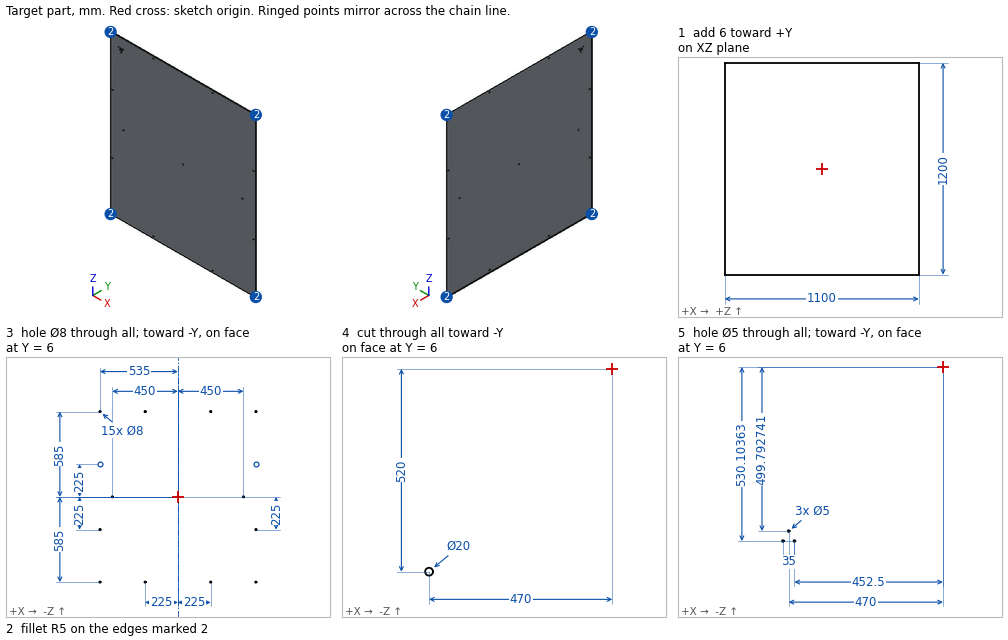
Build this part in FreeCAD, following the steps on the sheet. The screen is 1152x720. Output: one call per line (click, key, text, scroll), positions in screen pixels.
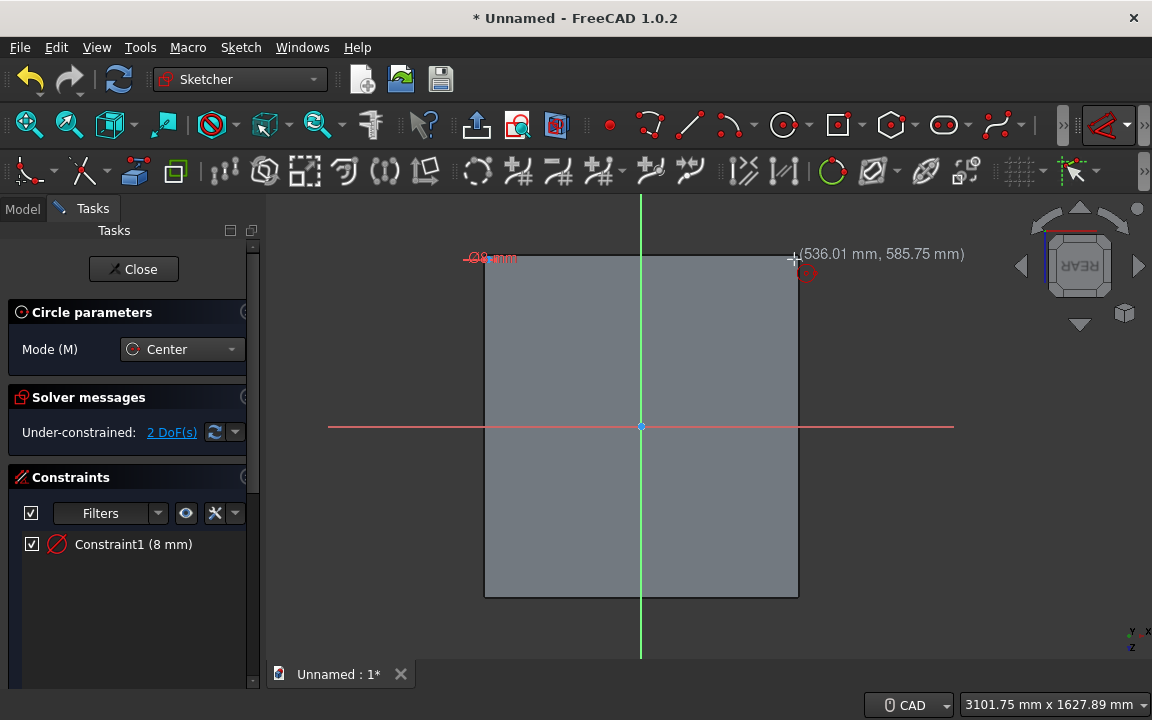
click(794, 259)
move(795, 259)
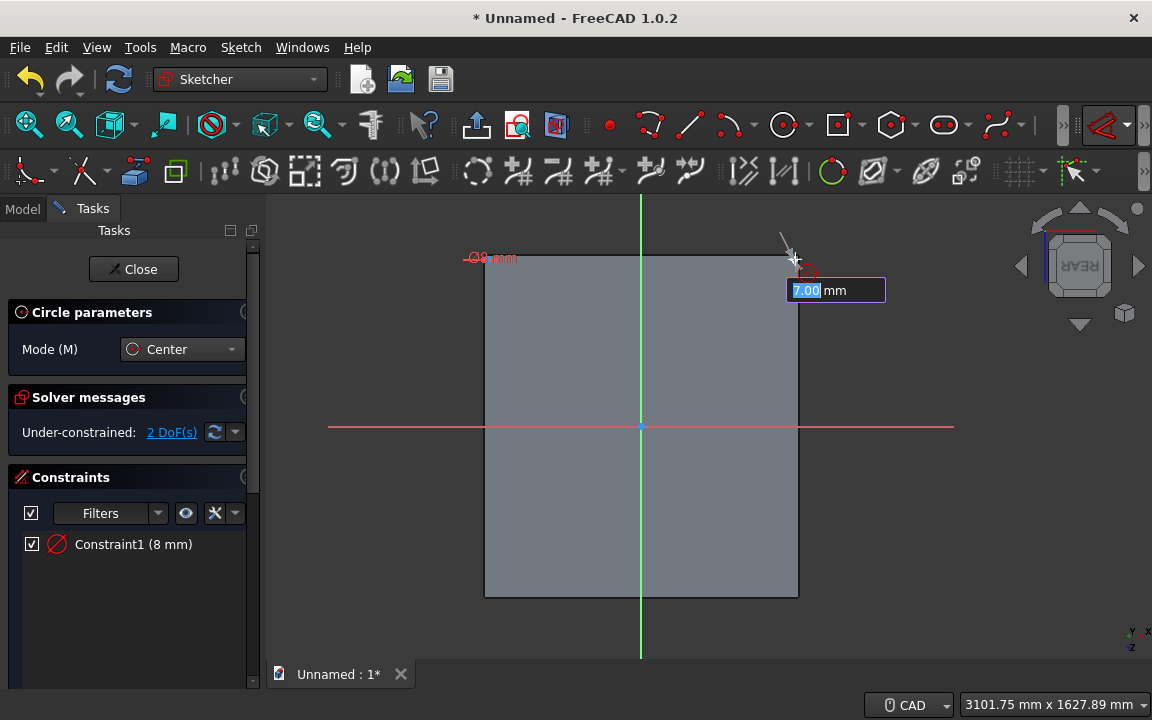
text(8)
key(Return)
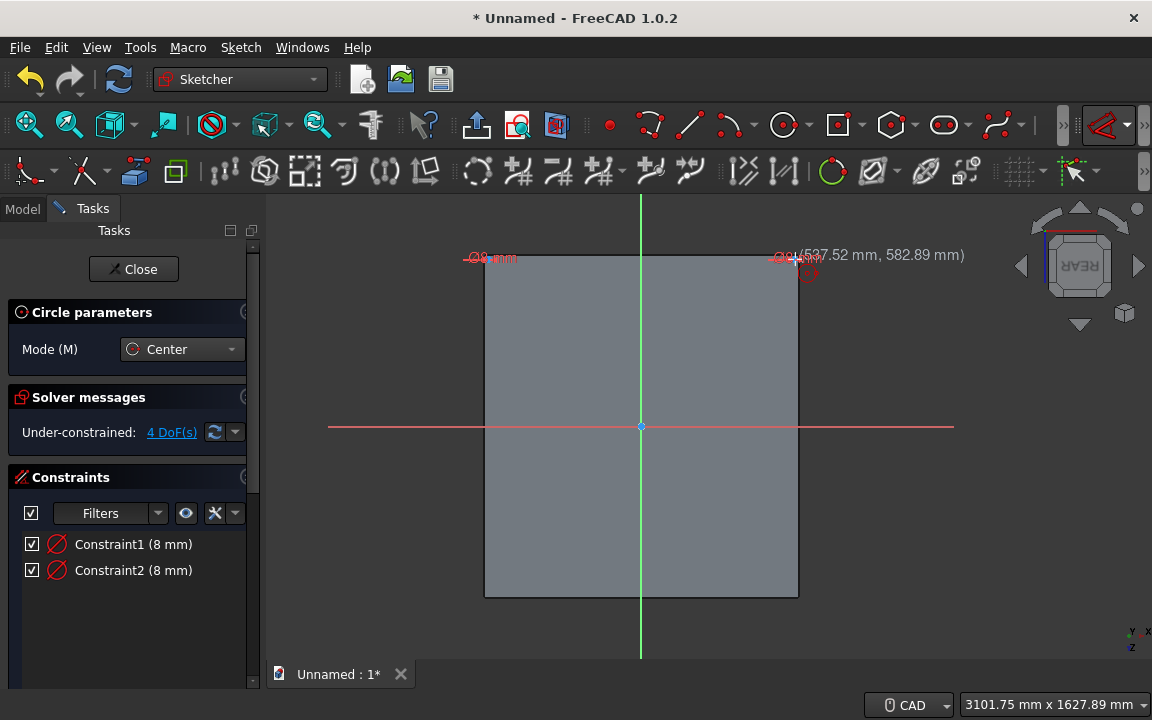
scroll(489, 594, up, 15)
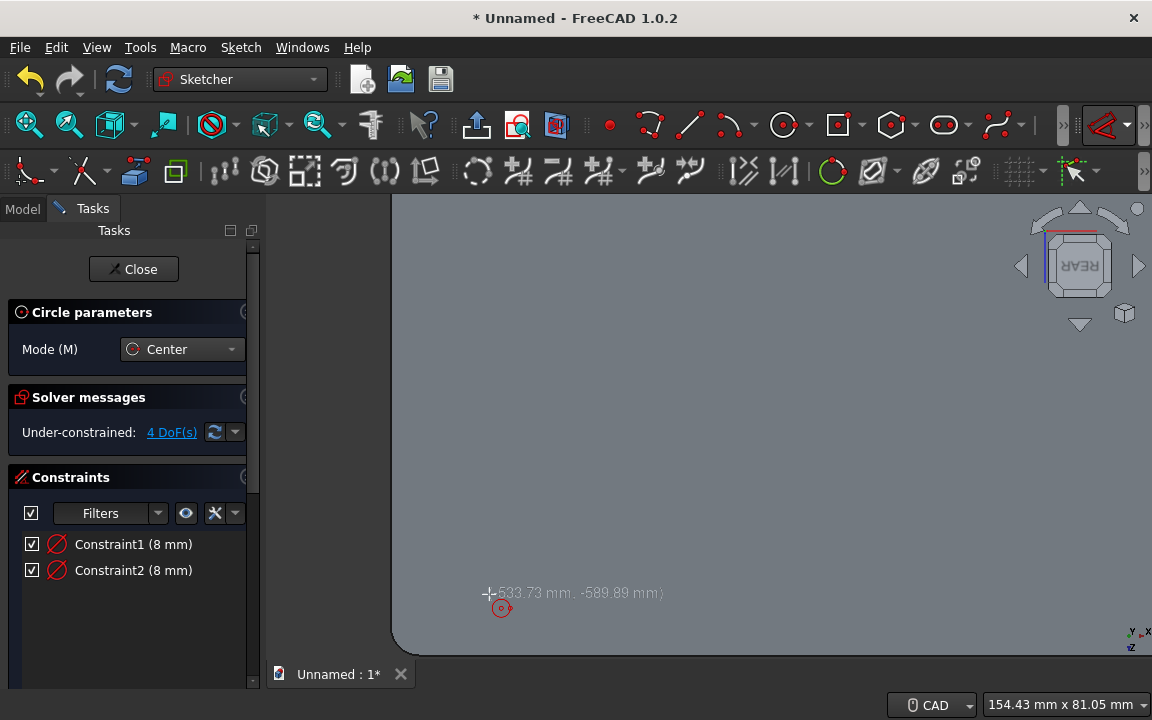
scroll(488, 595, down, 15)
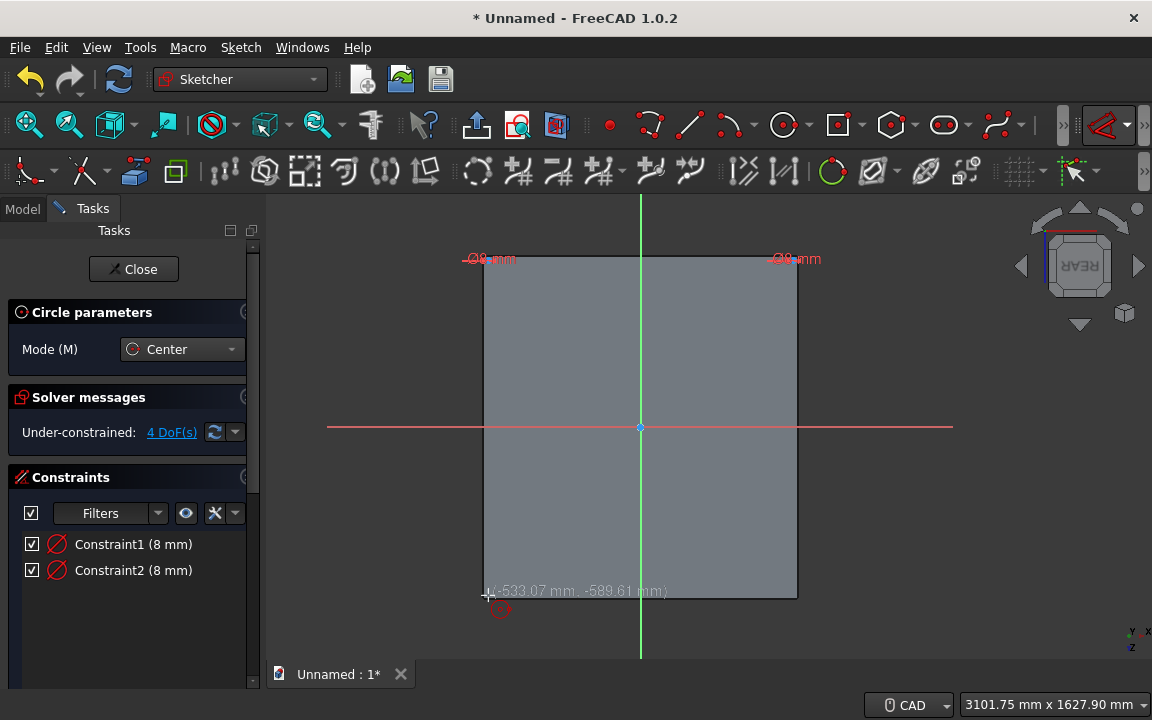
click(488, 595)
move(488, 594)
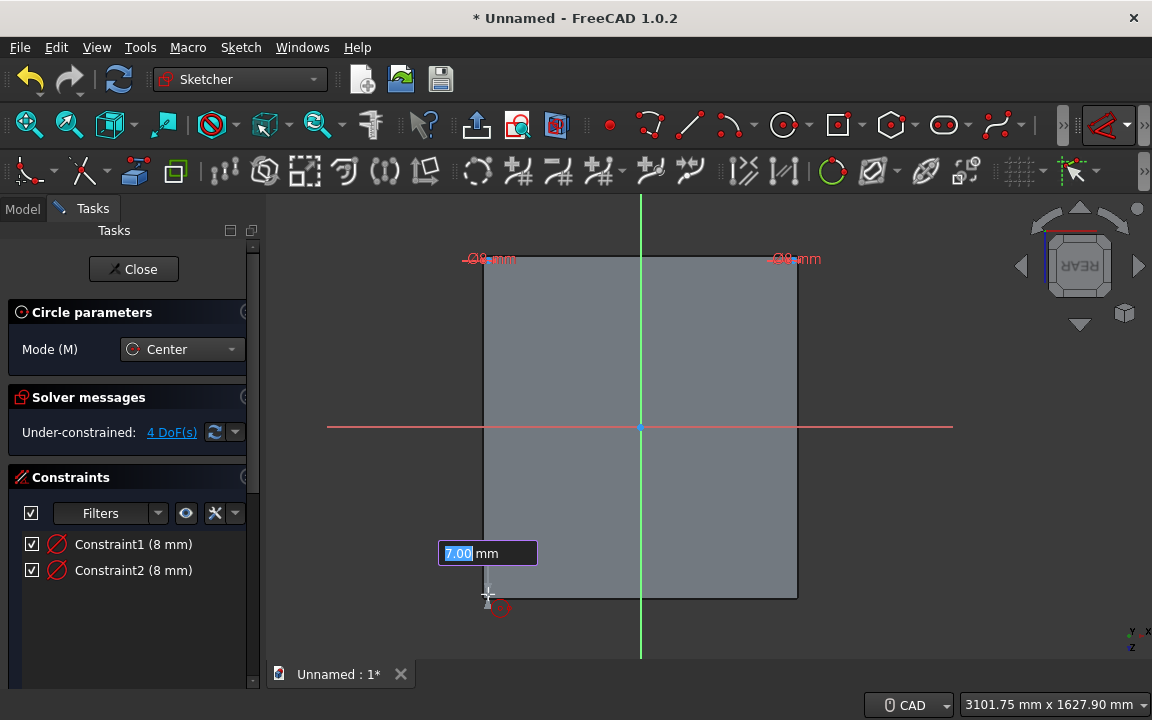
text(8)
key(Return)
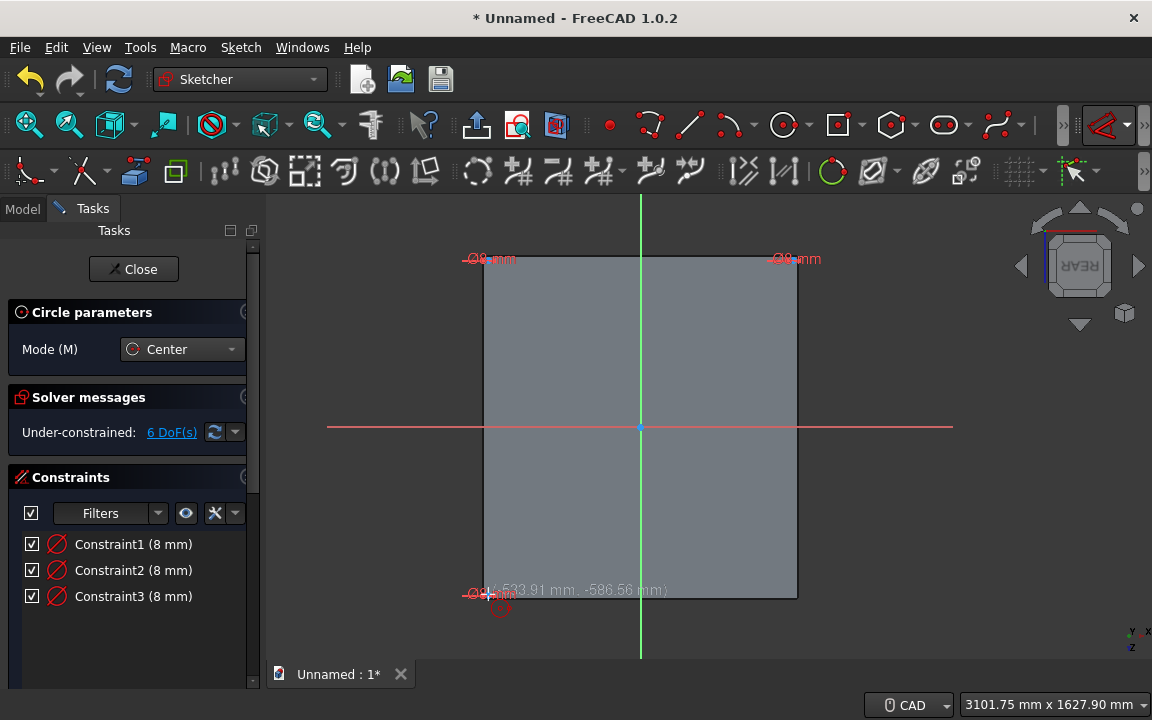
scroll(793, 595, up, 15)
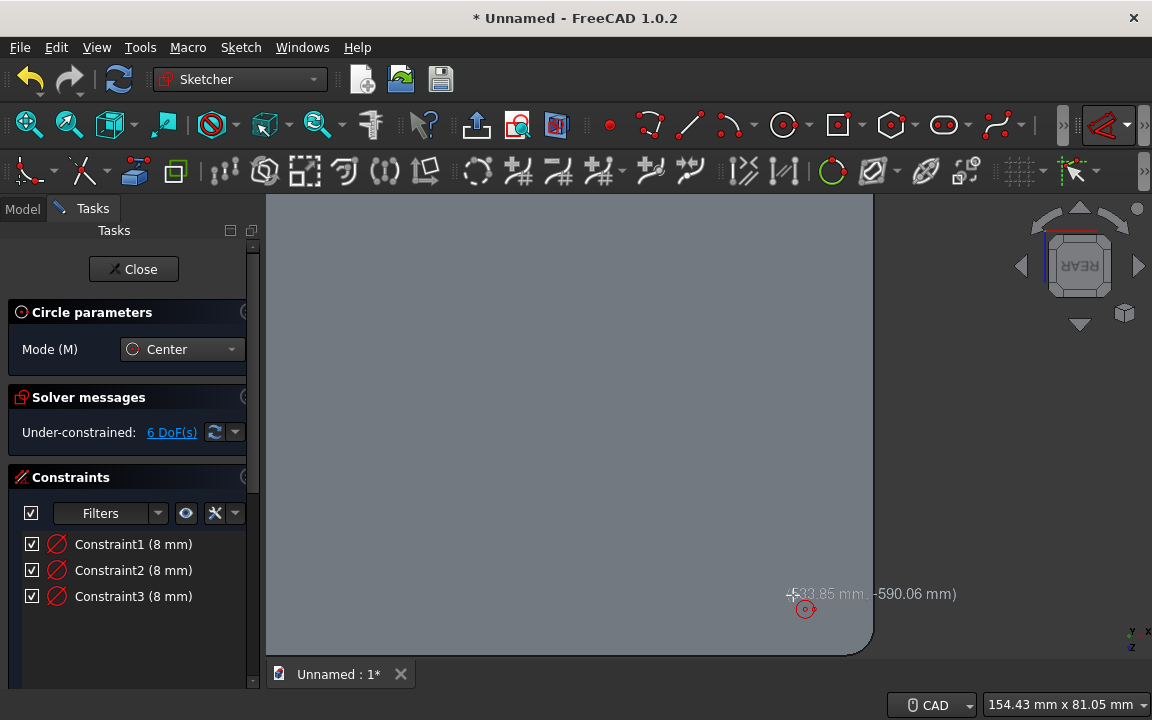
scroll(794, 595, down, 15)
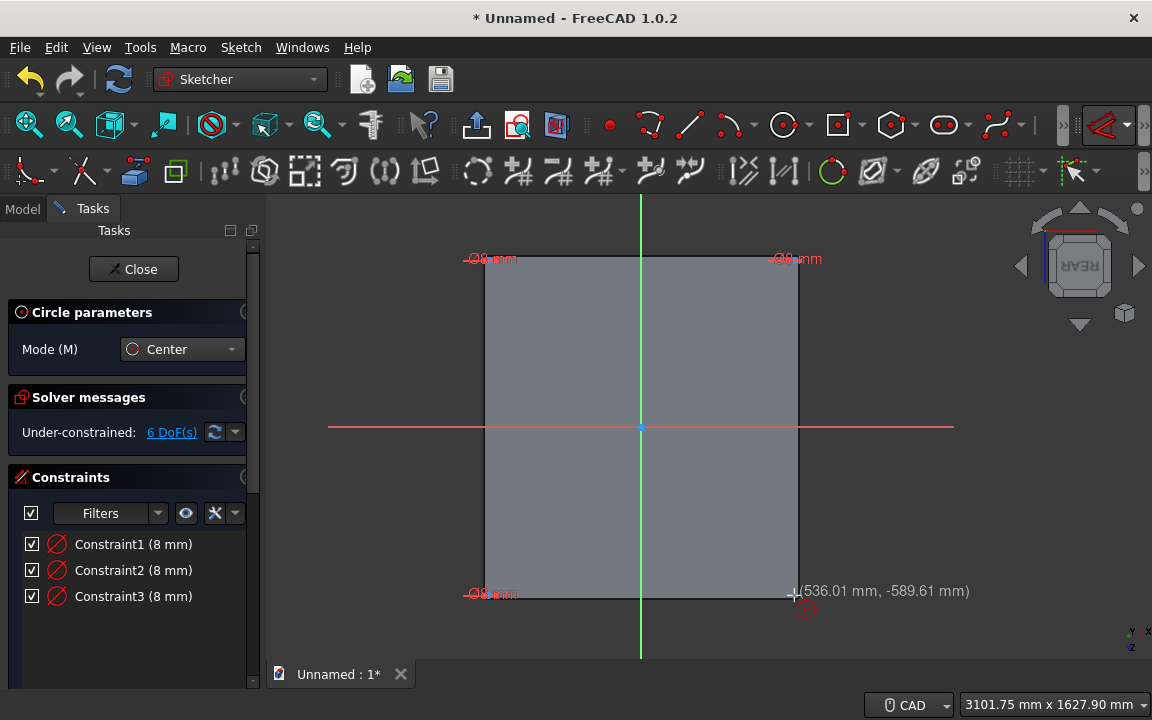
click(794, 595)
move(795, 594)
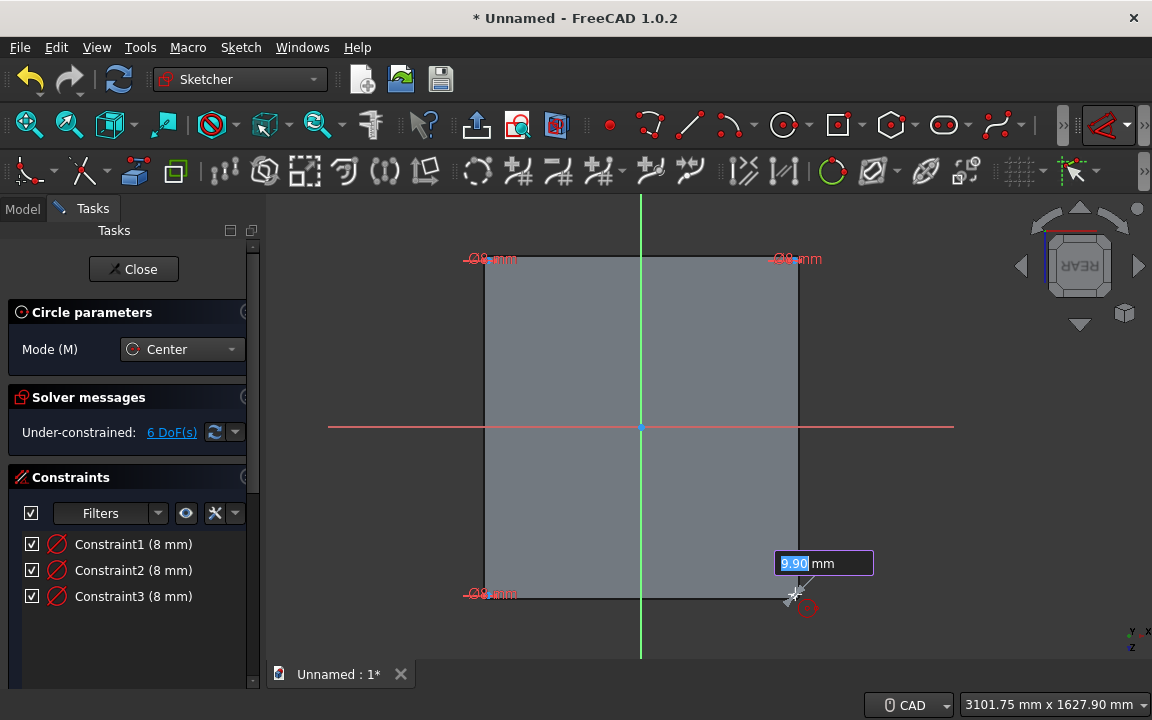
text(8)
key(Return)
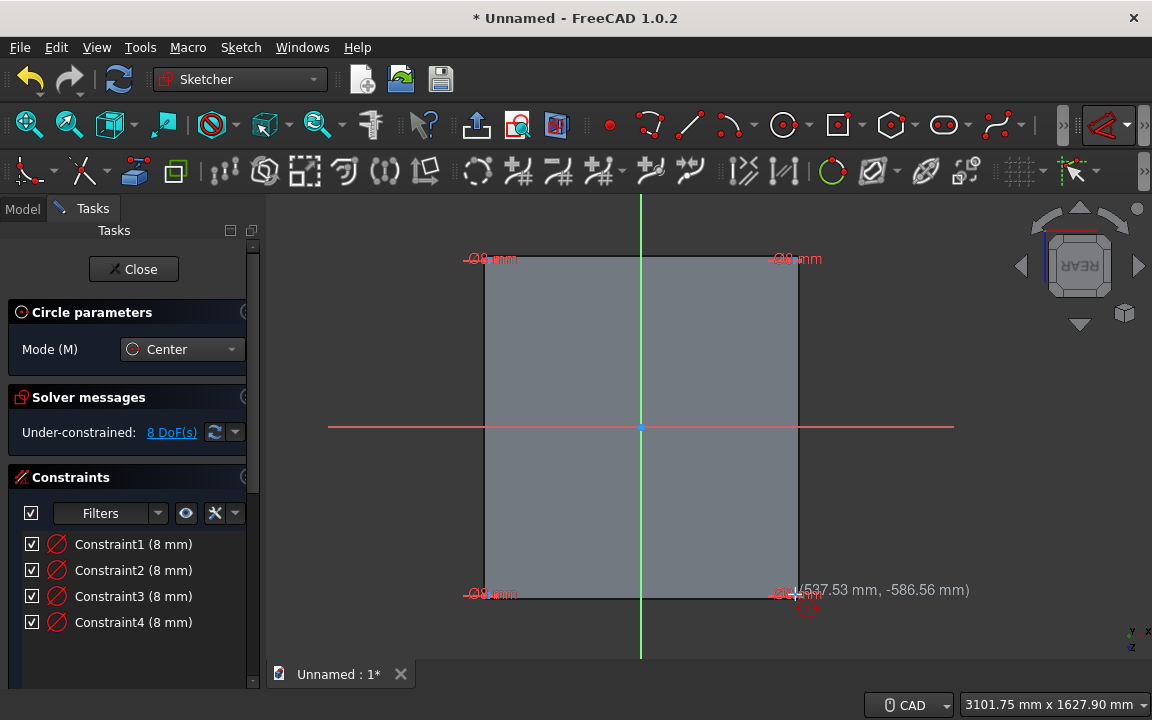
scroll(577, 595, up, 15)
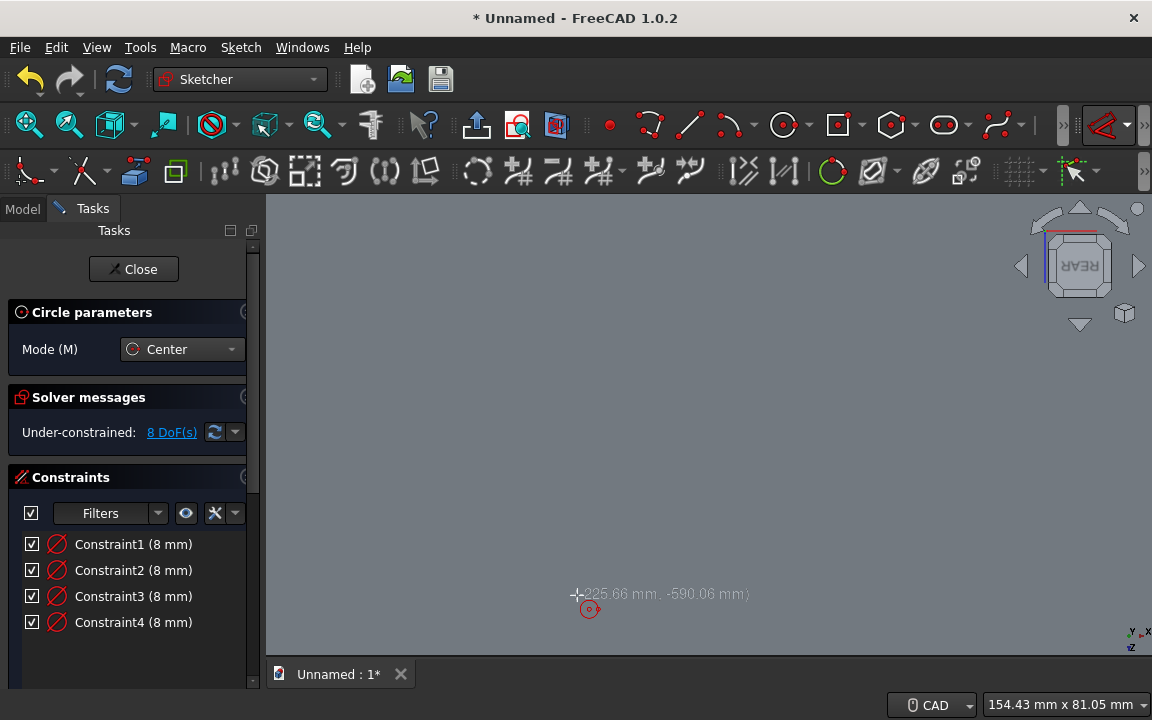
scroll(576, 595, down, 15)